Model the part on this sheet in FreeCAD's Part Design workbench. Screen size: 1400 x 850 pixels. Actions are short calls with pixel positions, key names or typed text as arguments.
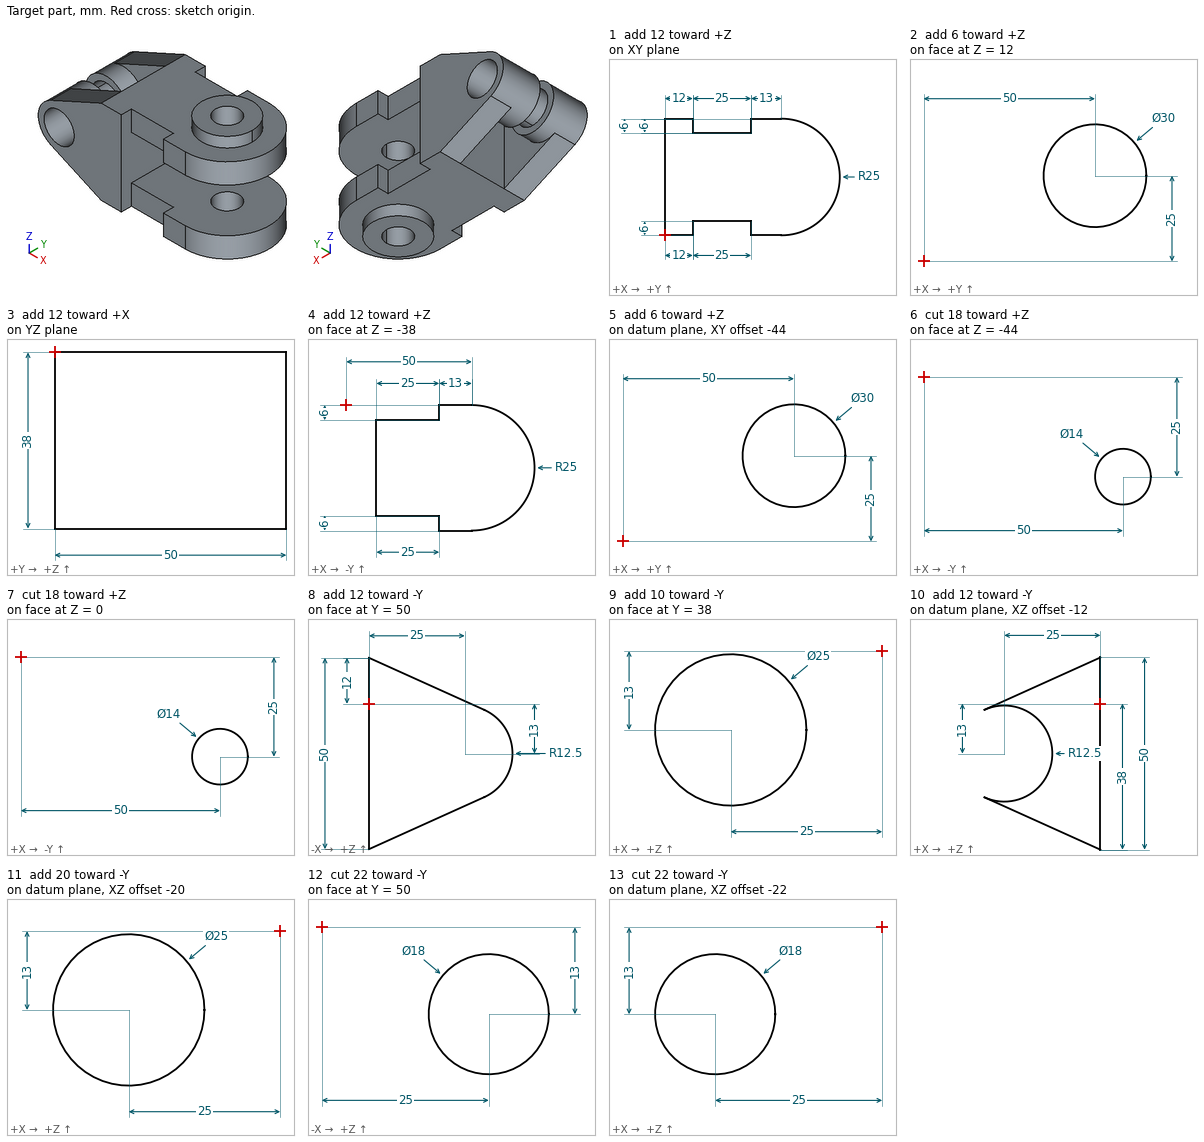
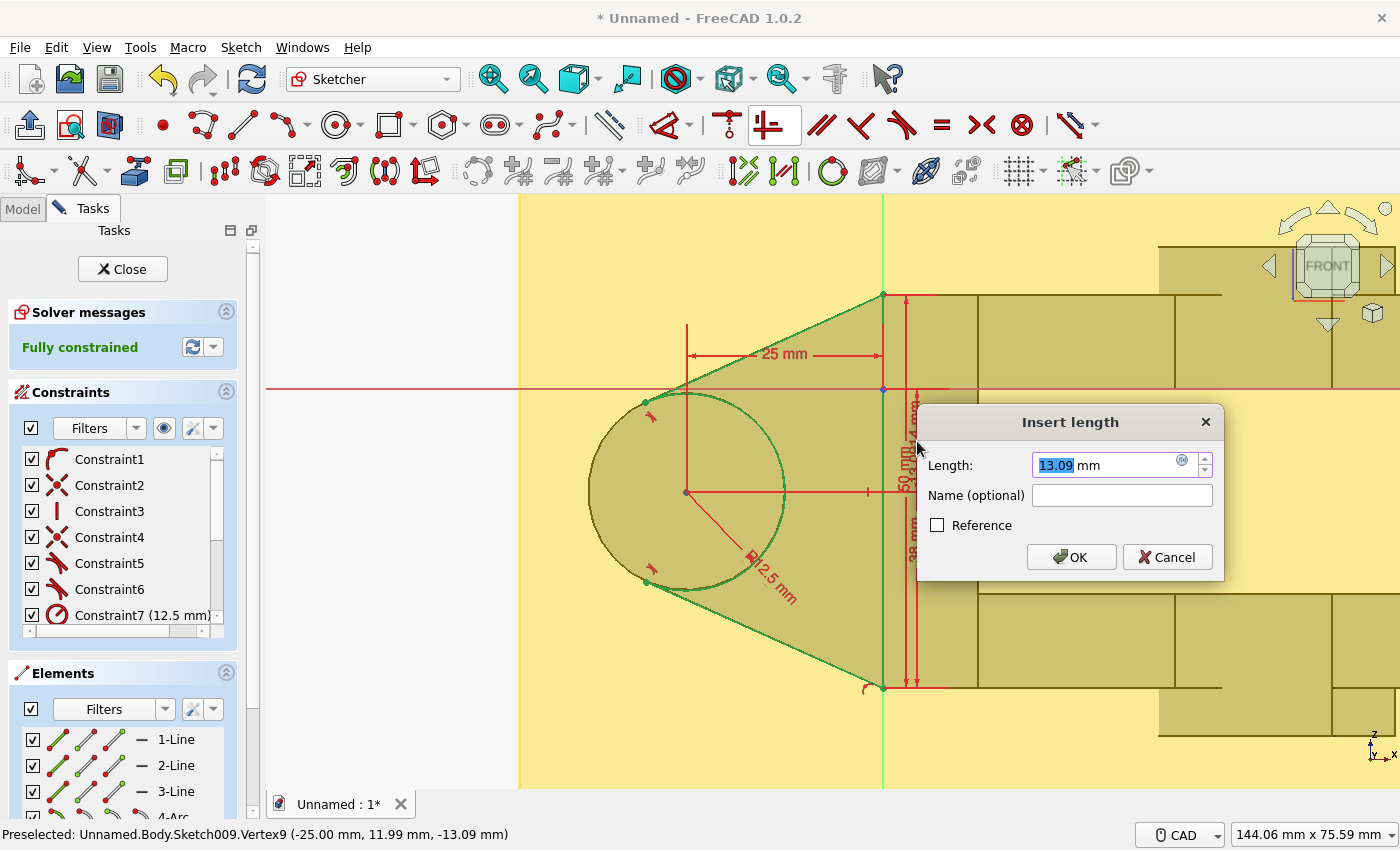
text(13)
key(Return)
key(Escape)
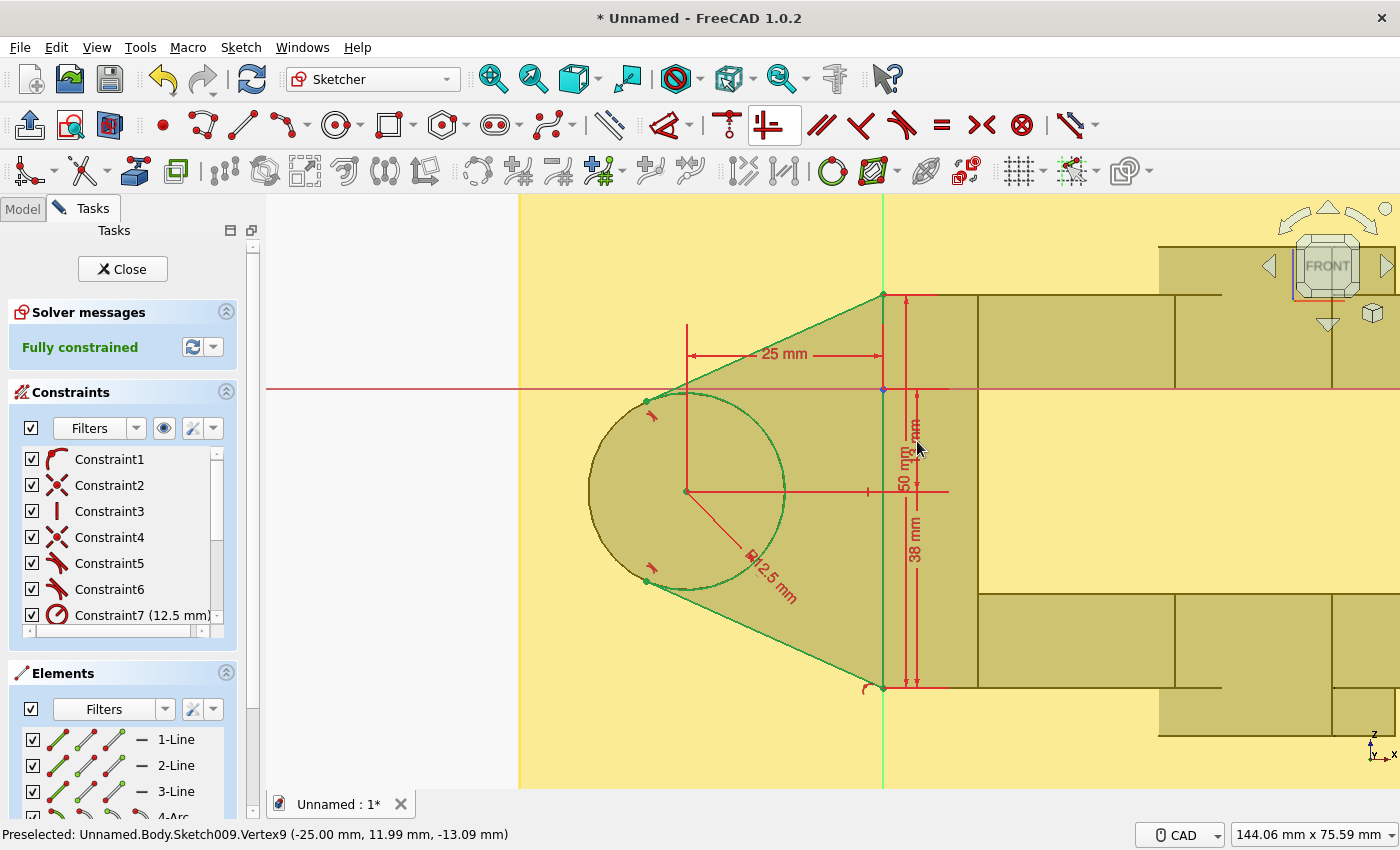
click(123, 269)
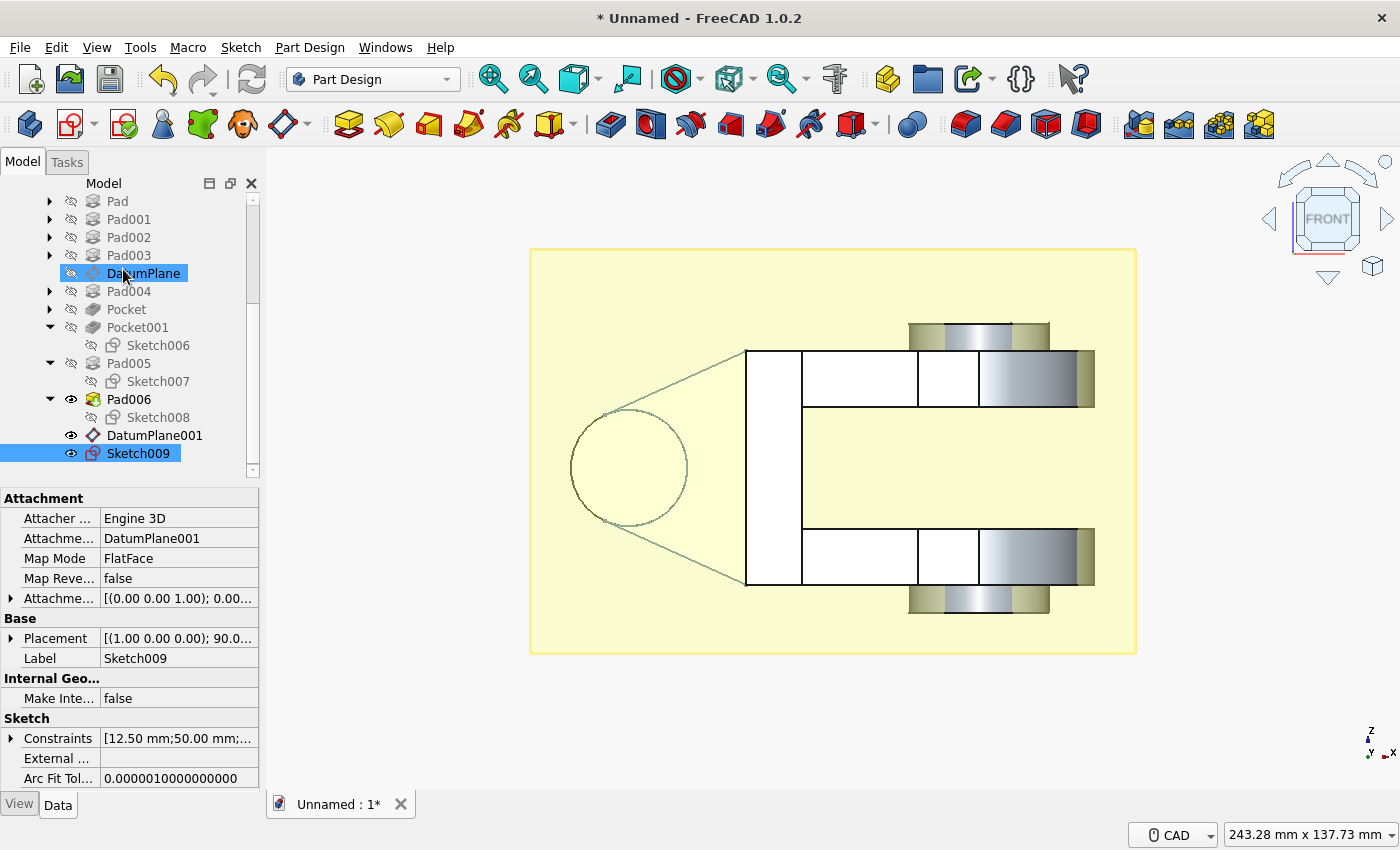
click(350, 124)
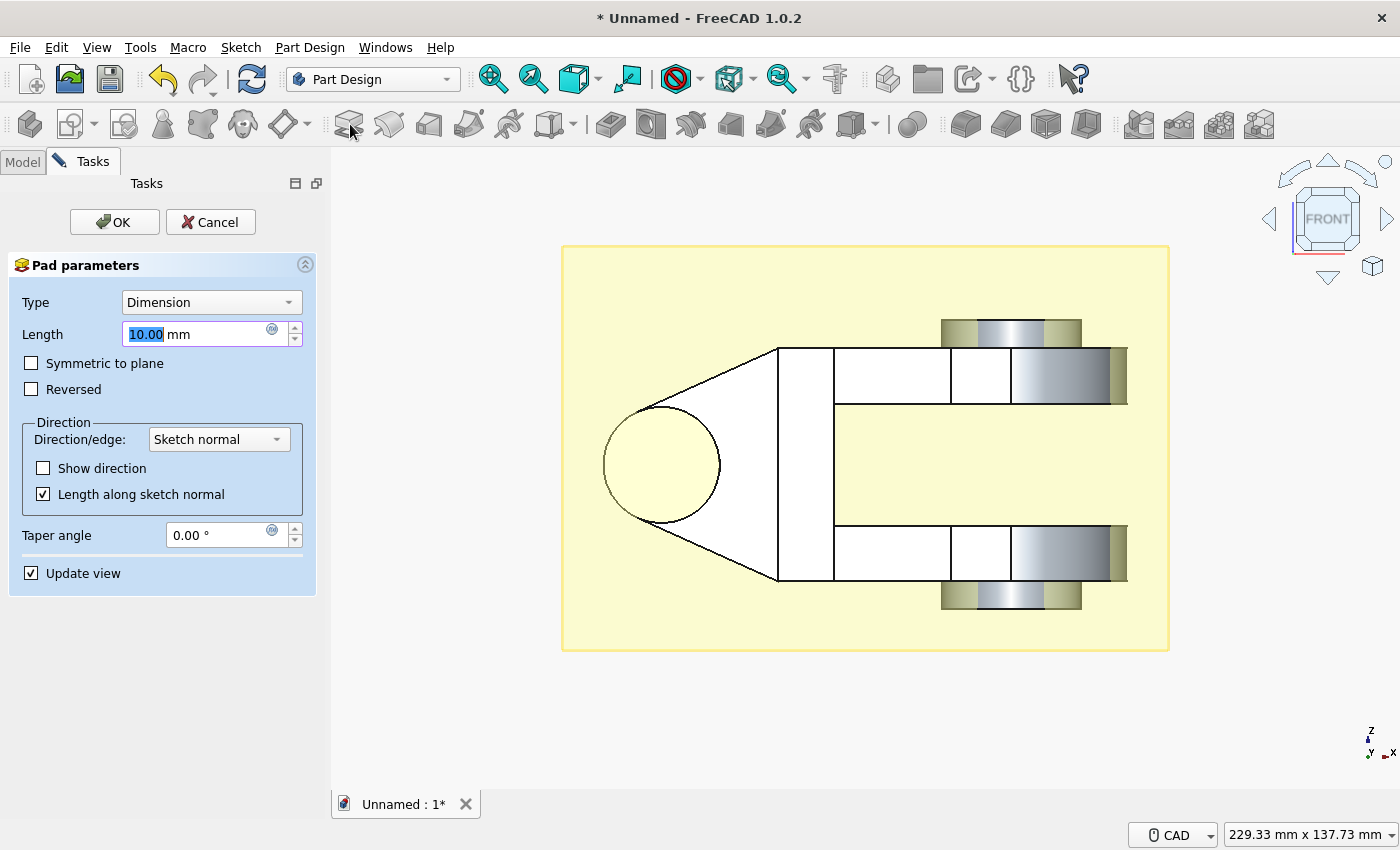
text(12)
key(Tab)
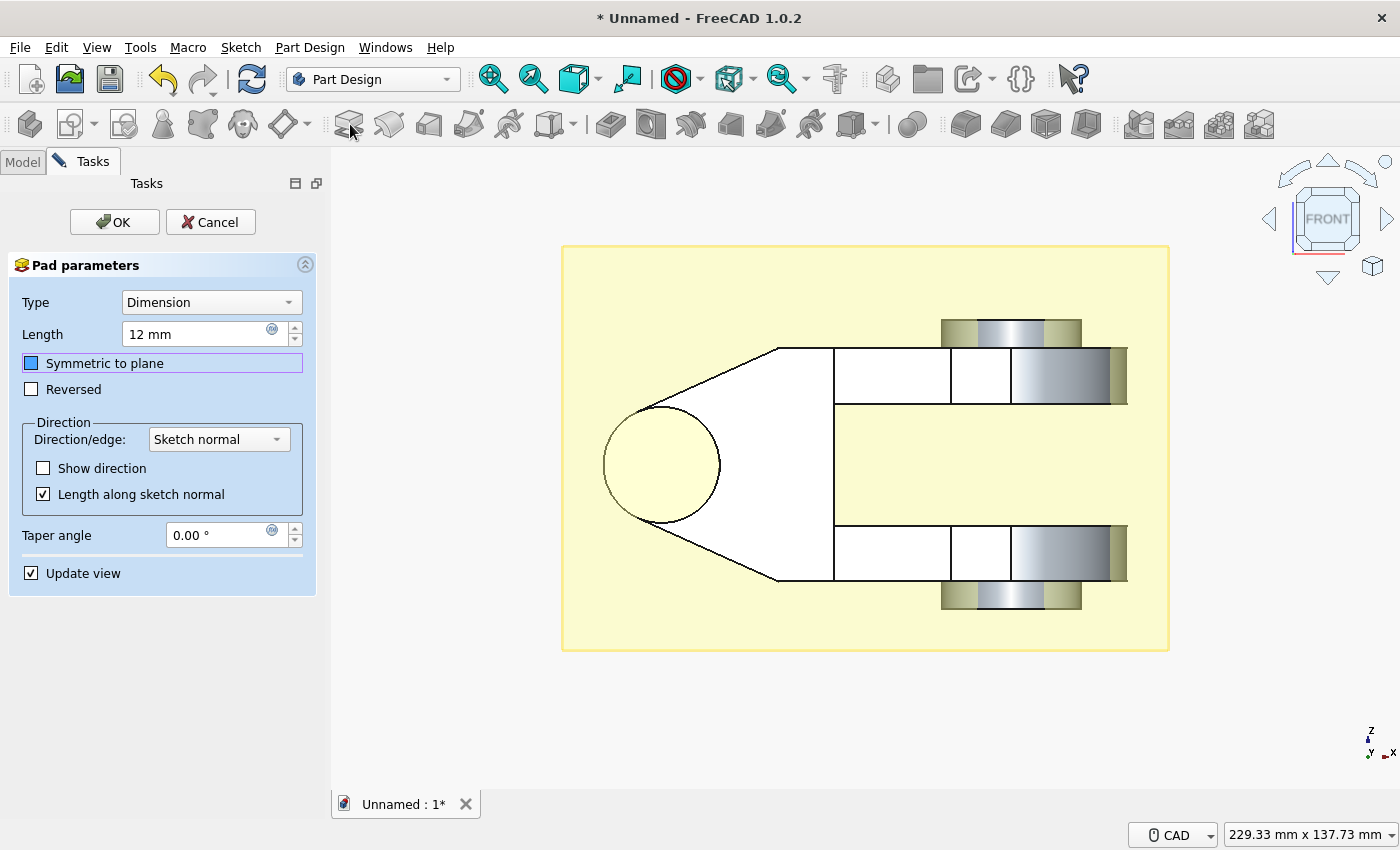
click(115, 222)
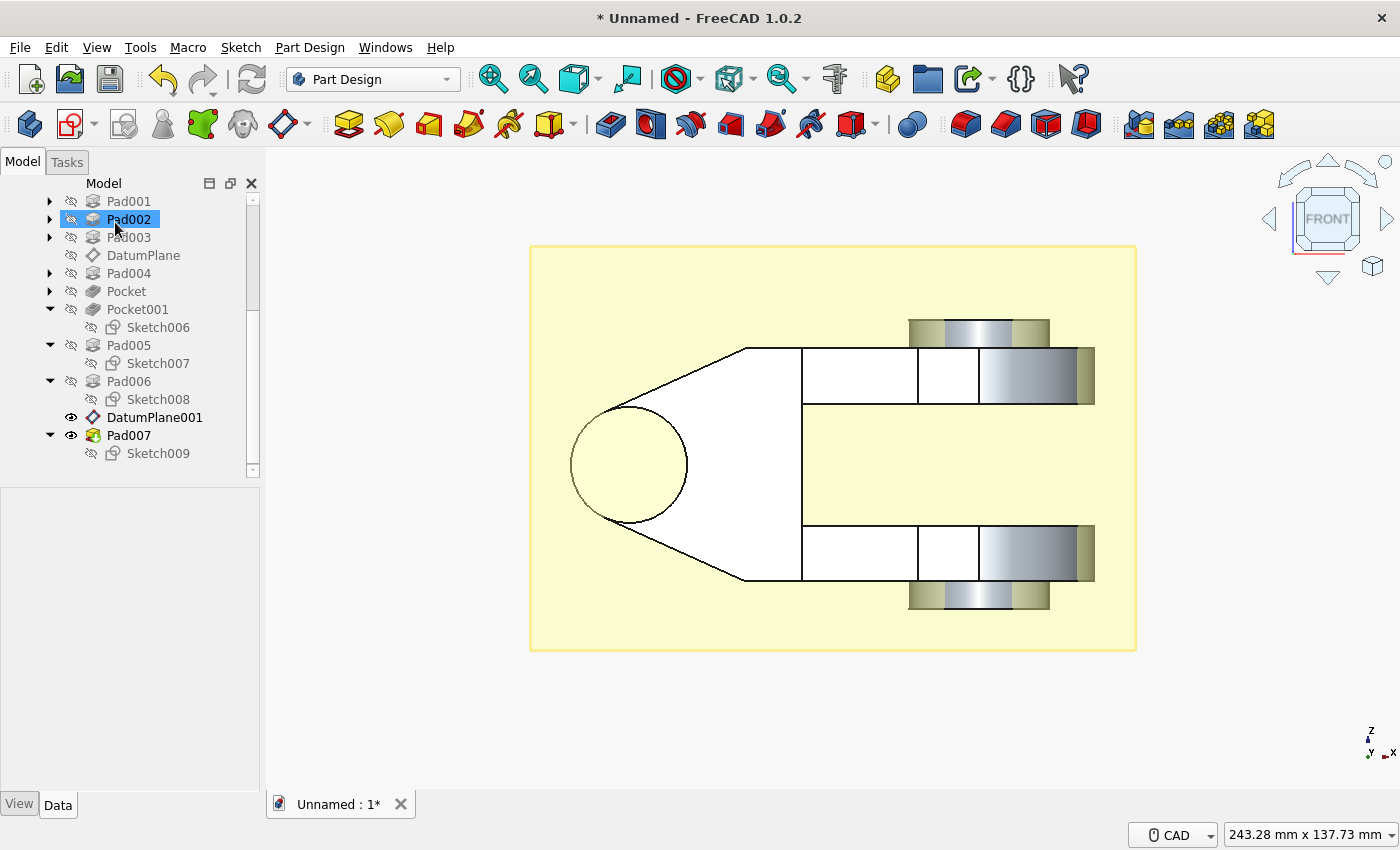
click(116, 417)
key(space)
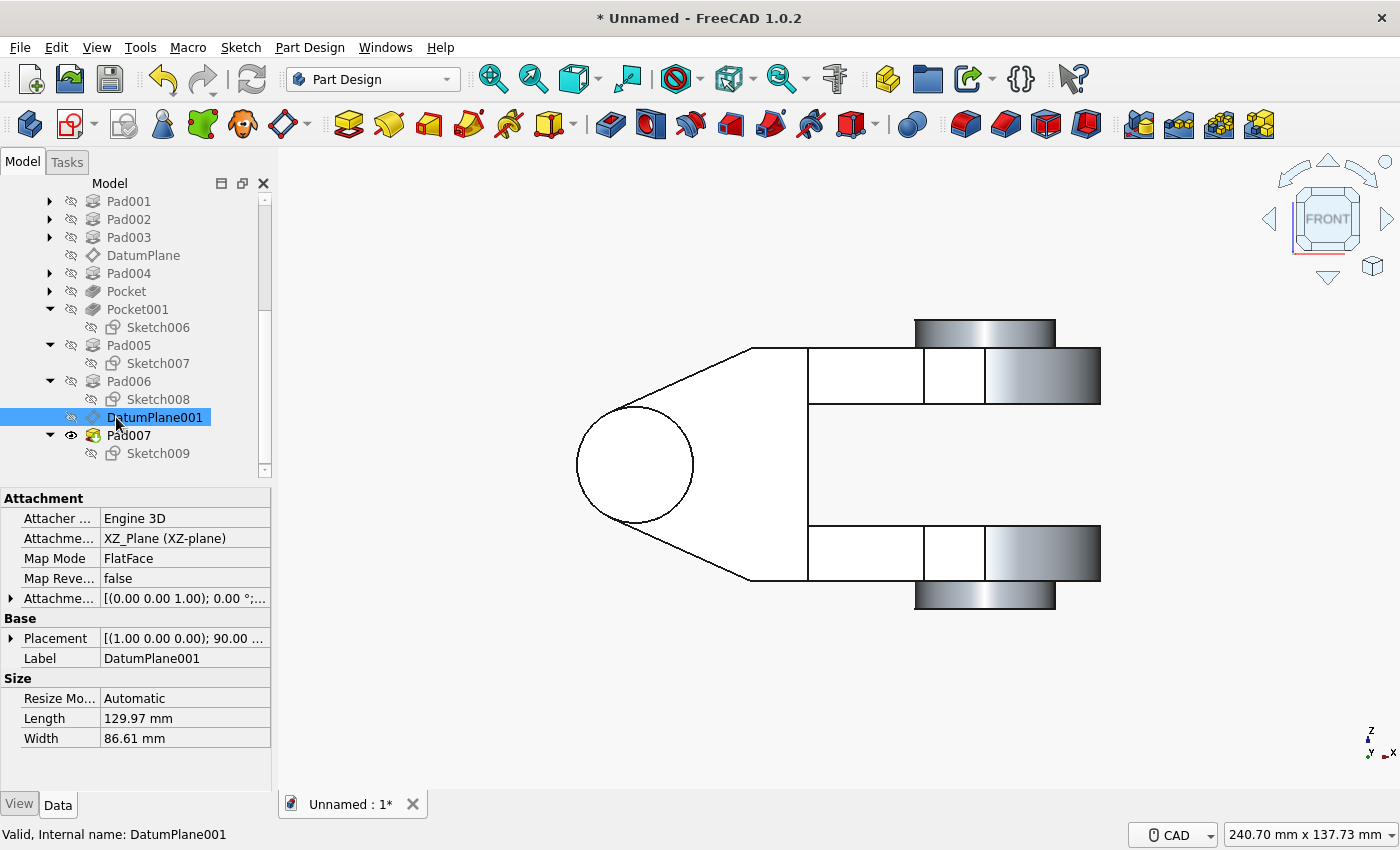
scroll(140, 323, down, 3)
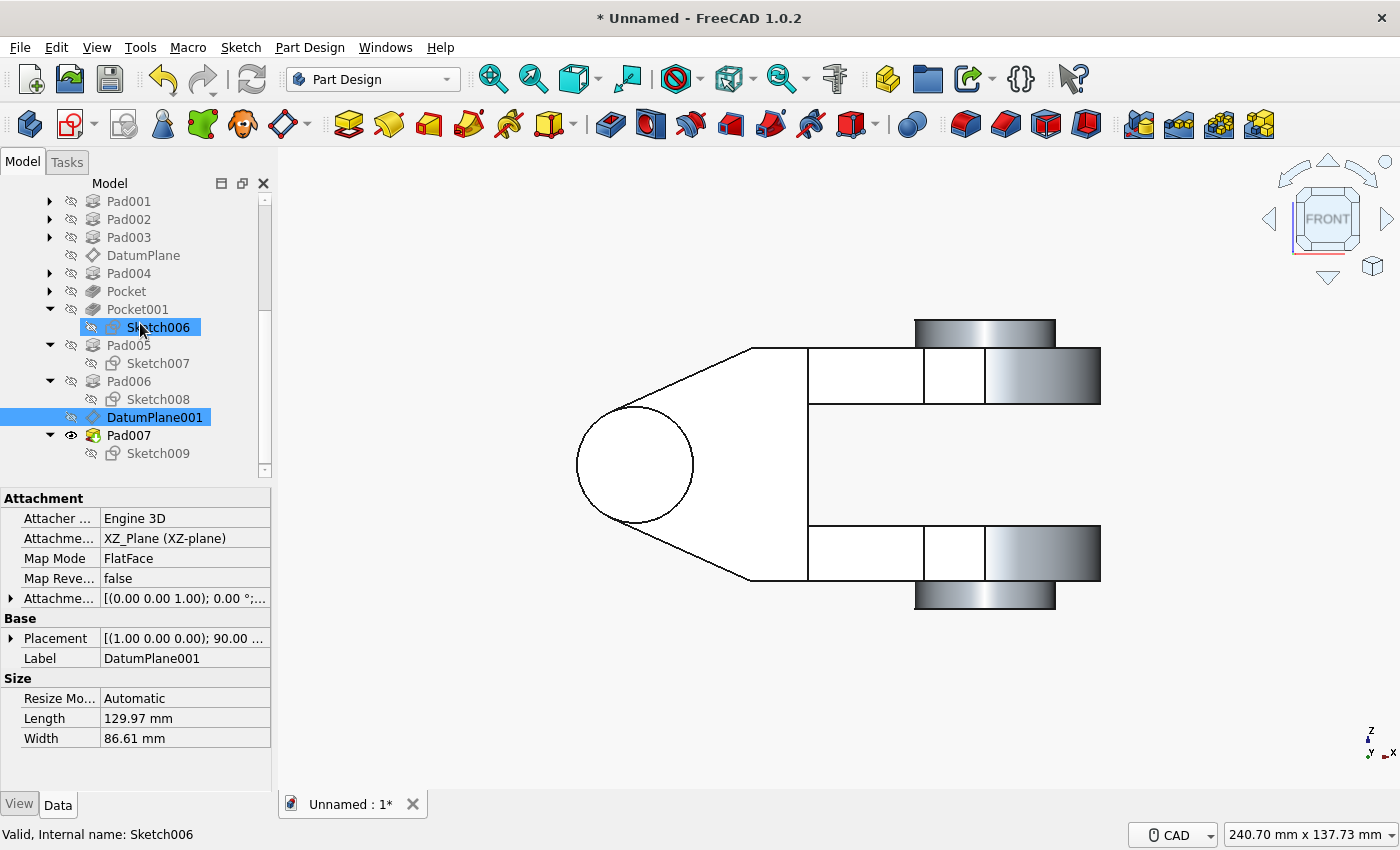
scroll(140, 323, up, 15)